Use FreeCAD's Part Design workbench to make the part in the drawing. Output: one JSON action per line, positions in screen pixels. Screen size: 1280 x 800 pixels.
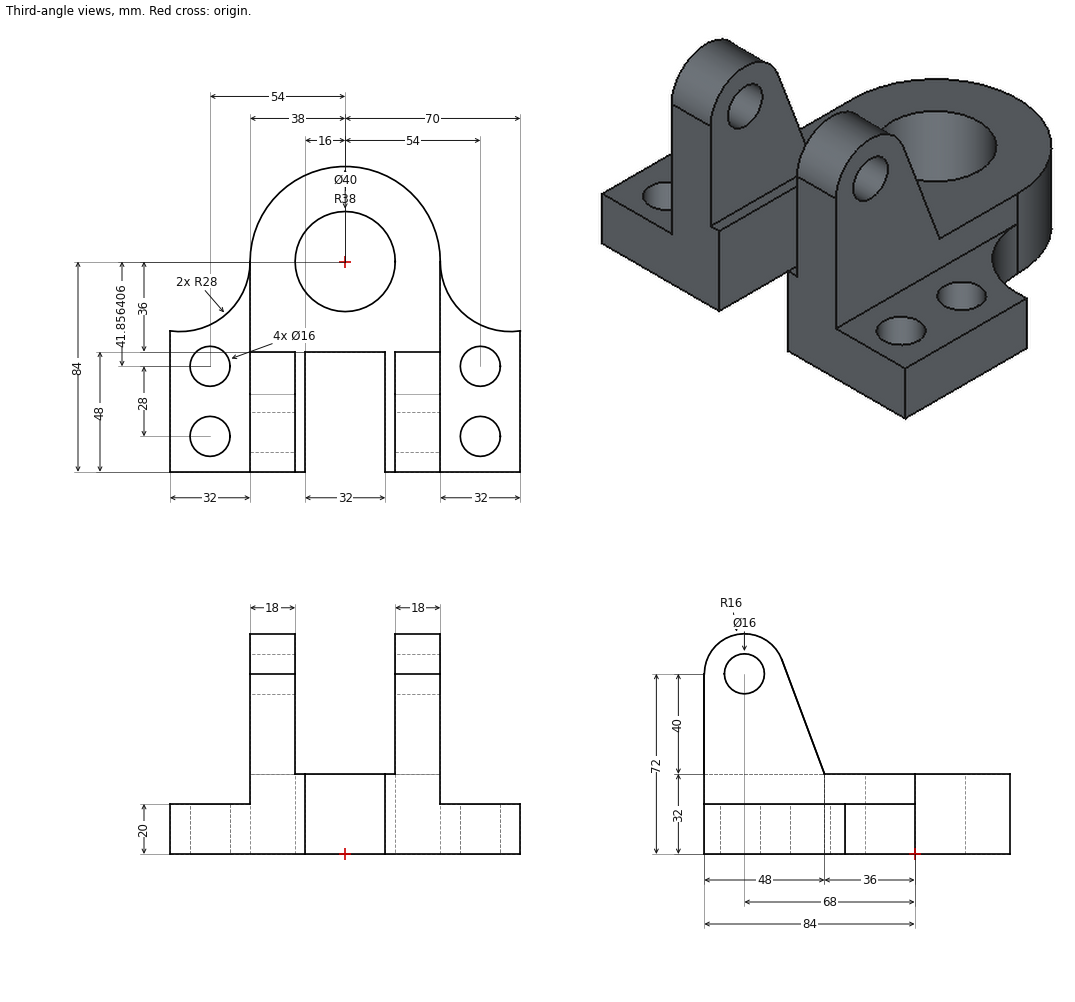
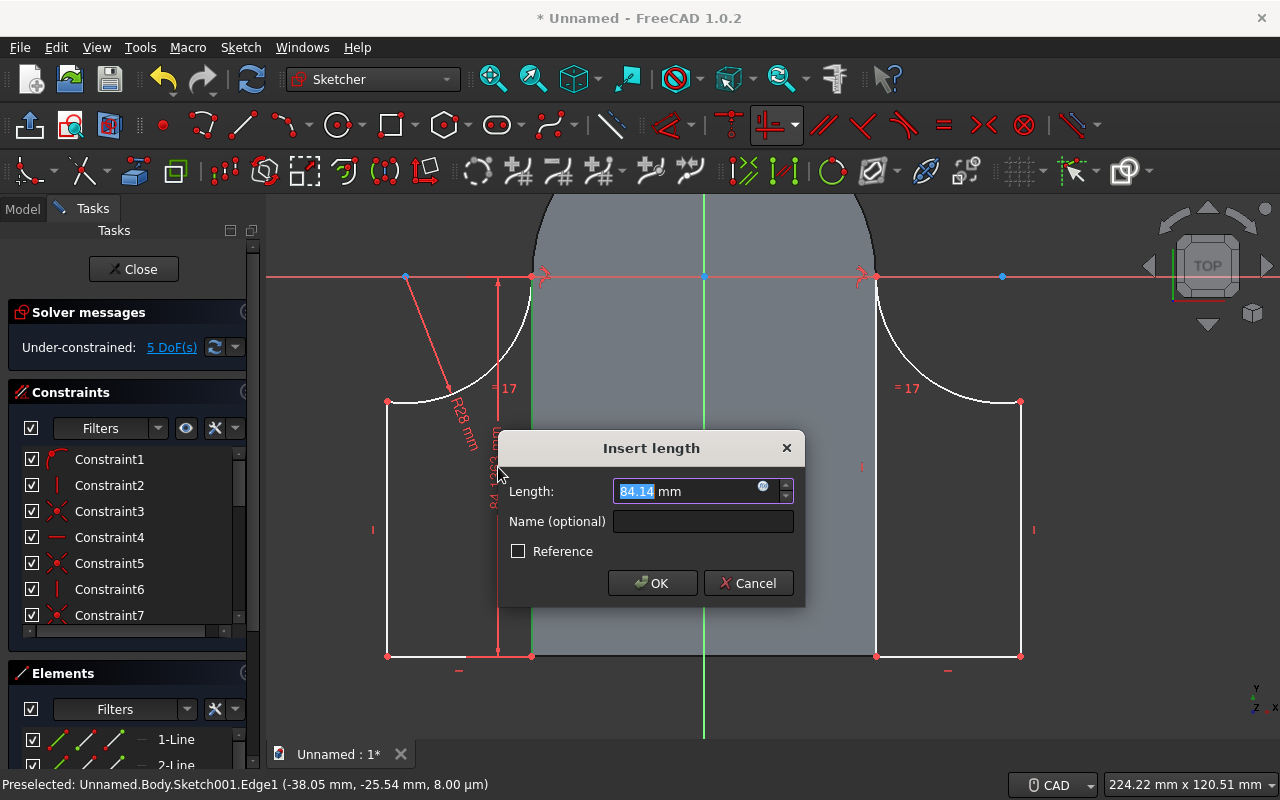
{"action": "type", "text": "84"}
{"action": "key", "text": "Return"}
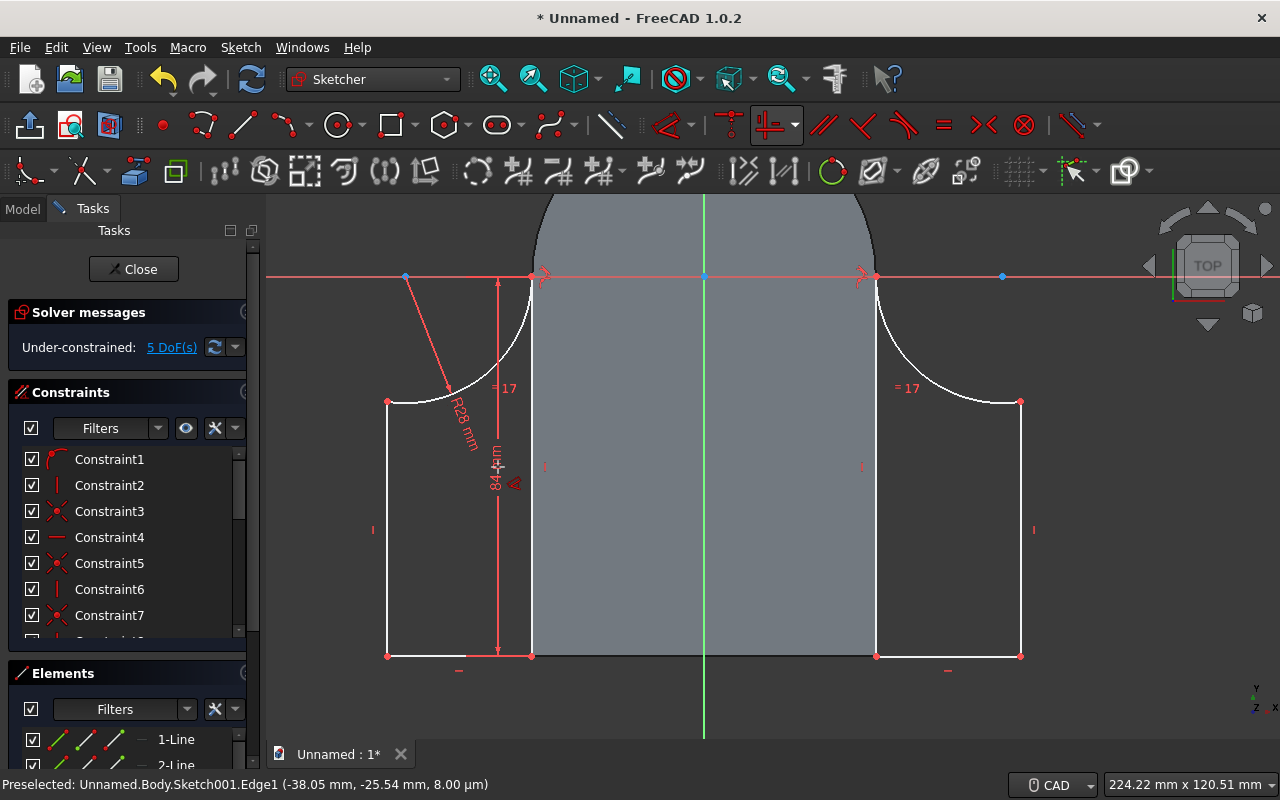
{"action": "left_click", "coordinate": [488, 656]}
{"action": "left_click", "coordinate": [459, 690]}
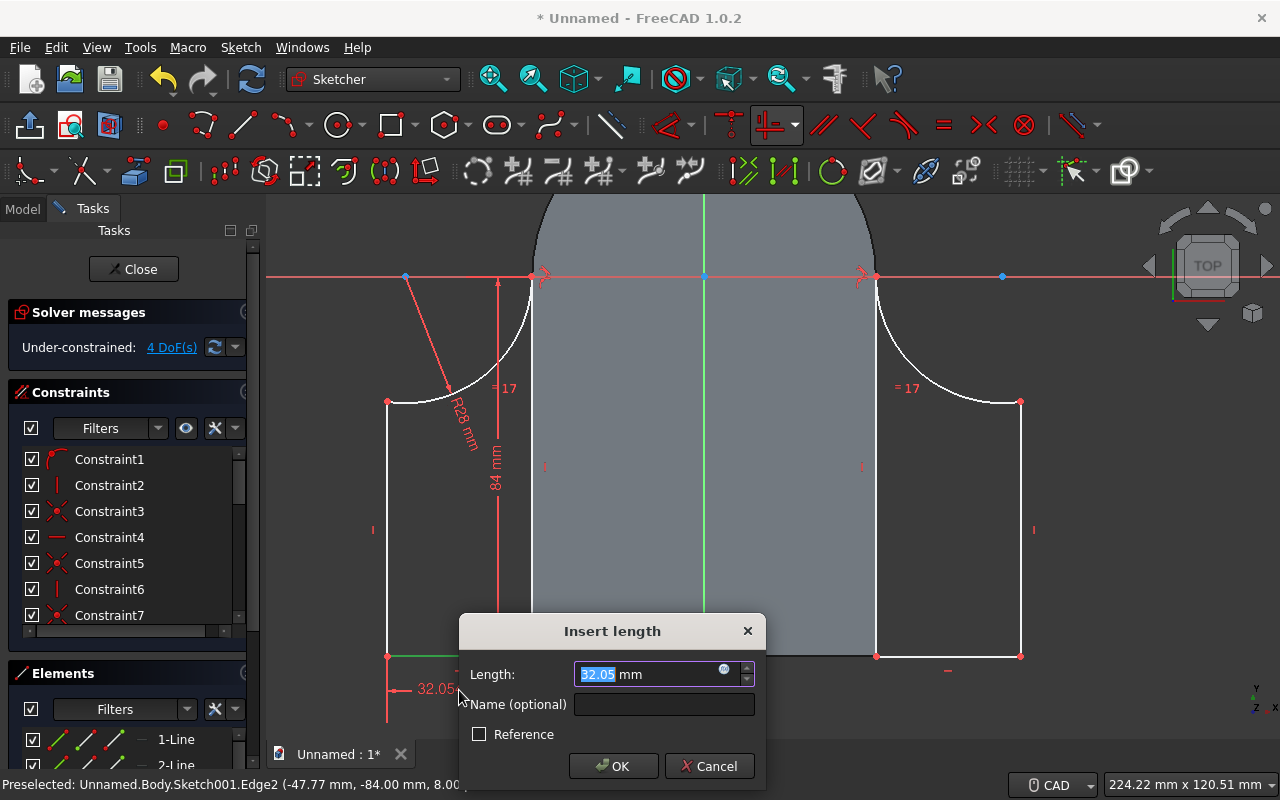
{"action": "type", "text": "32"}
{"action": "key", "text": "Return"}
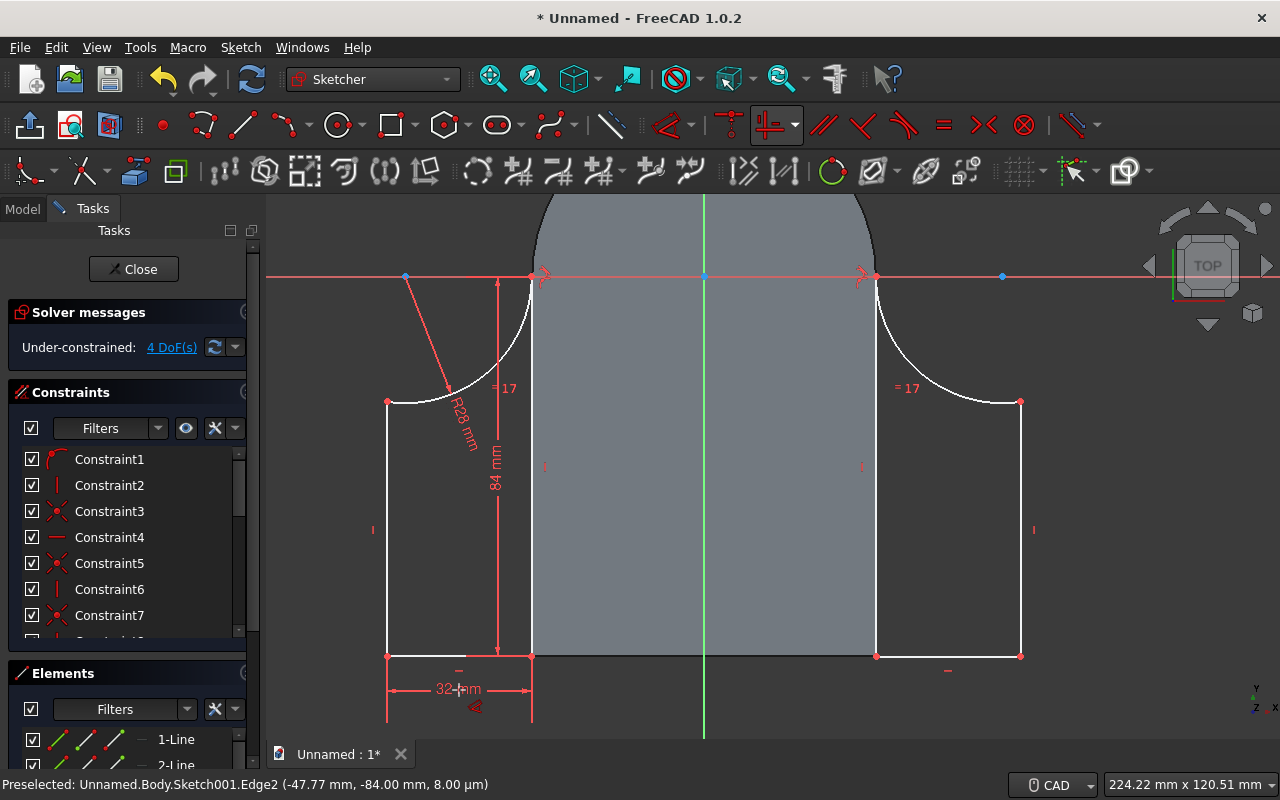
{"action": "left_click", "coordinate": [978, 657]}
{"action": "left_click", "coordinate": [949, 691]}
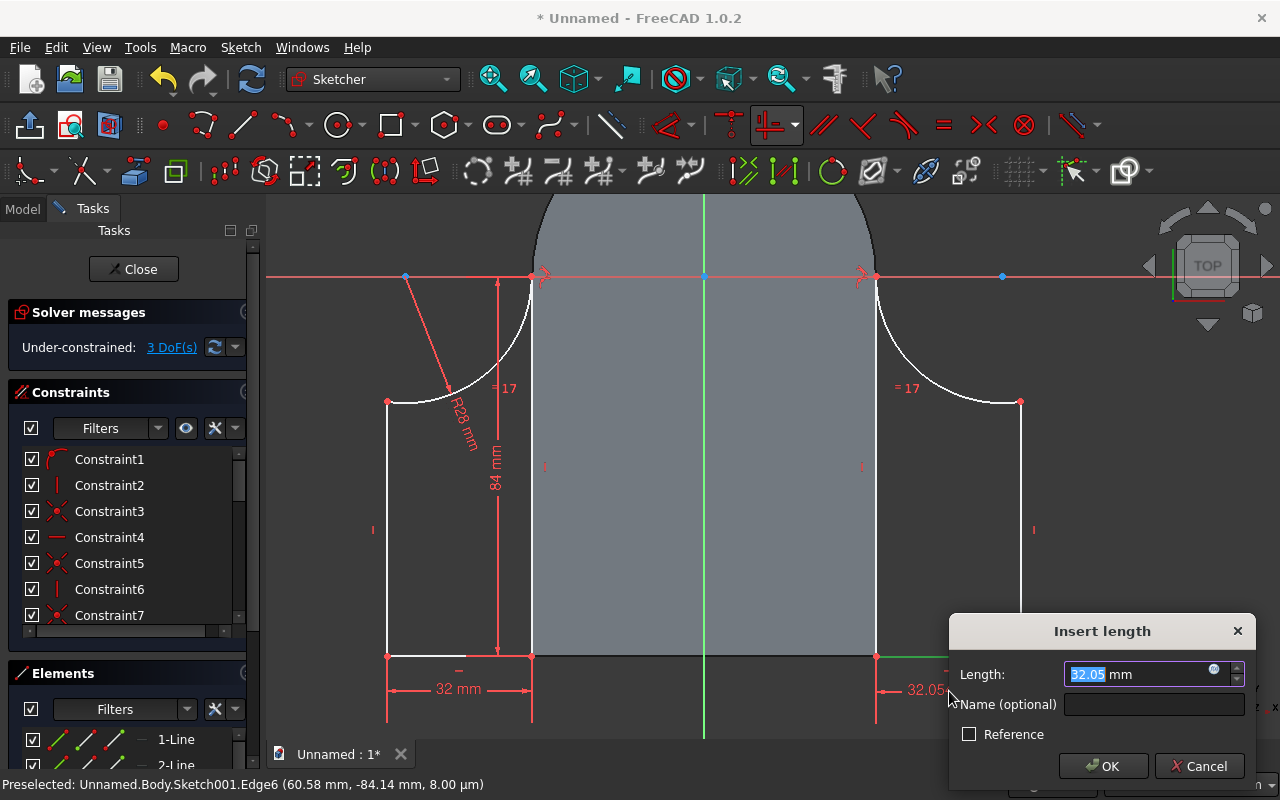
{"action": "type", "text": "32"}
{"action": "key", "text": "Return"}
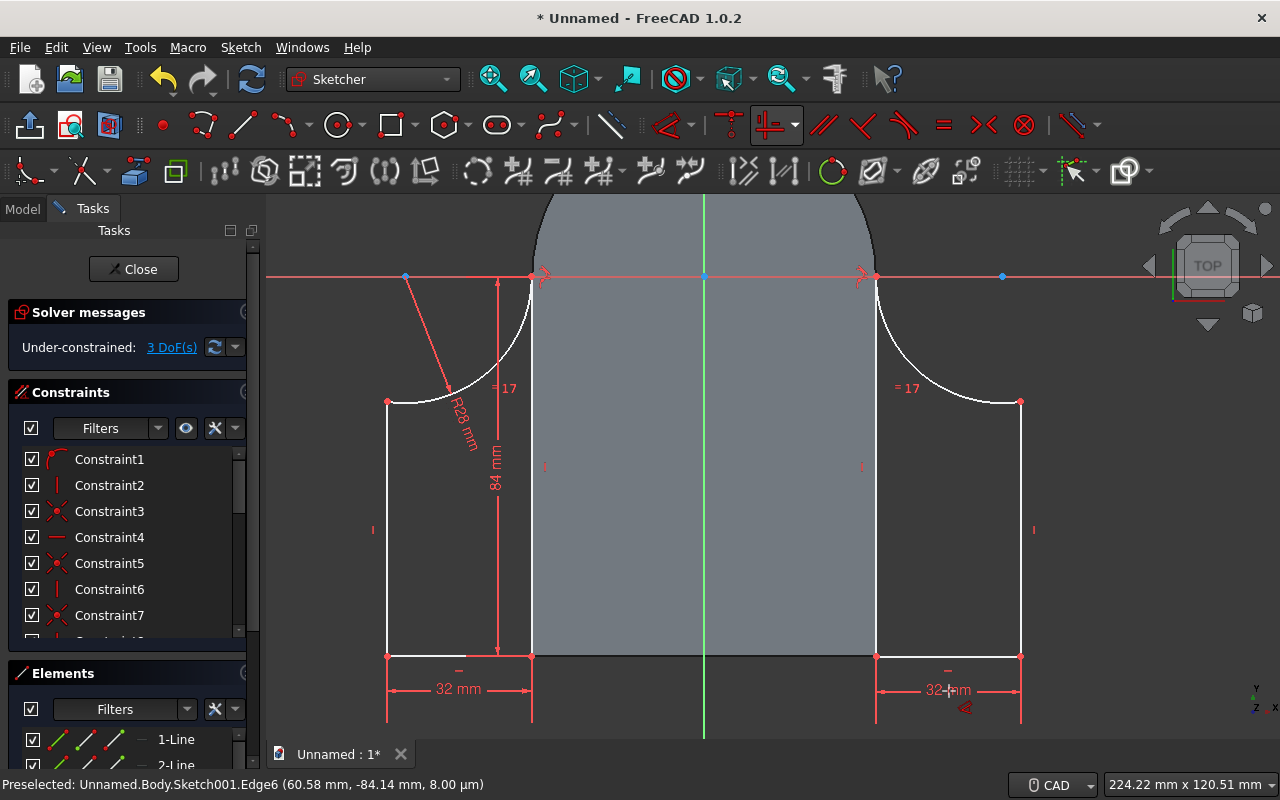
{"action": "left_click", "coordinate": [876, 543]}
{"action": "left_click", "coordinate": [910, 467]}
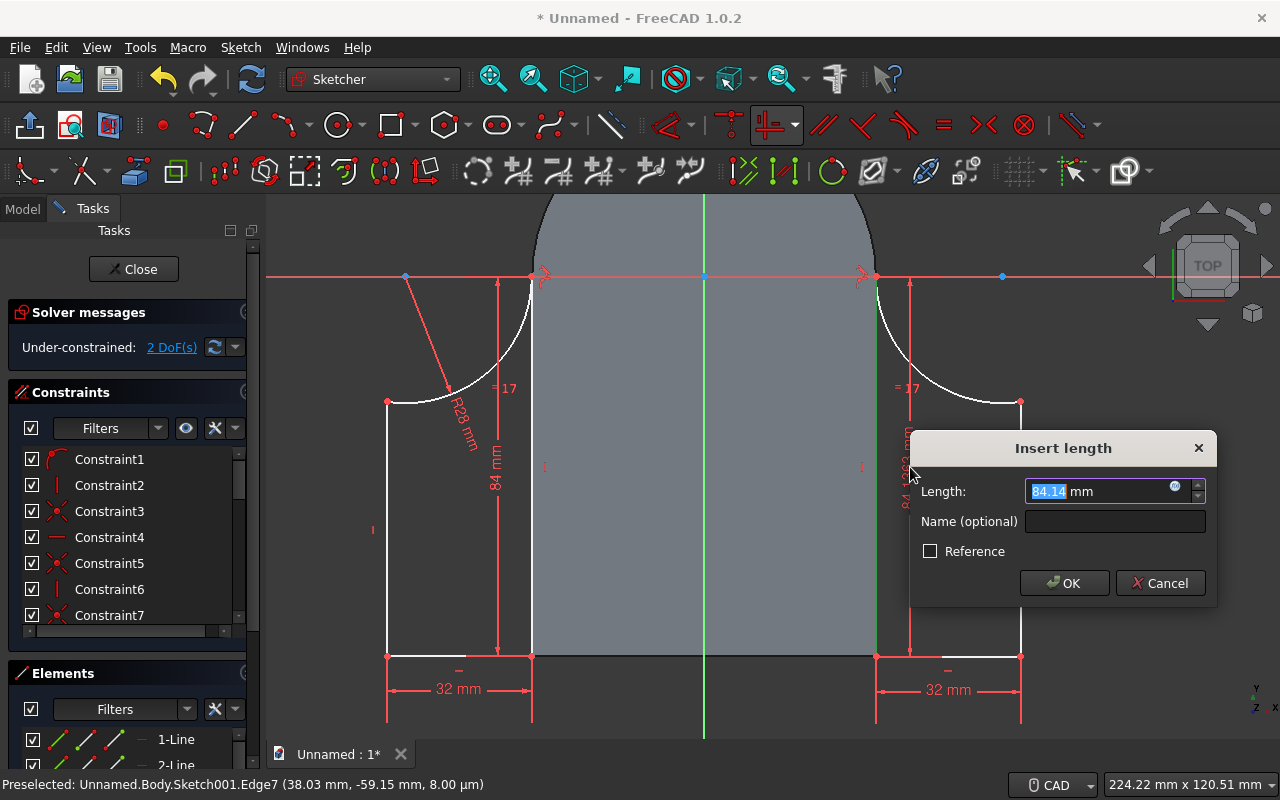
{"action": "type", "text": "84"}
{"action": "key", "text": "Return"}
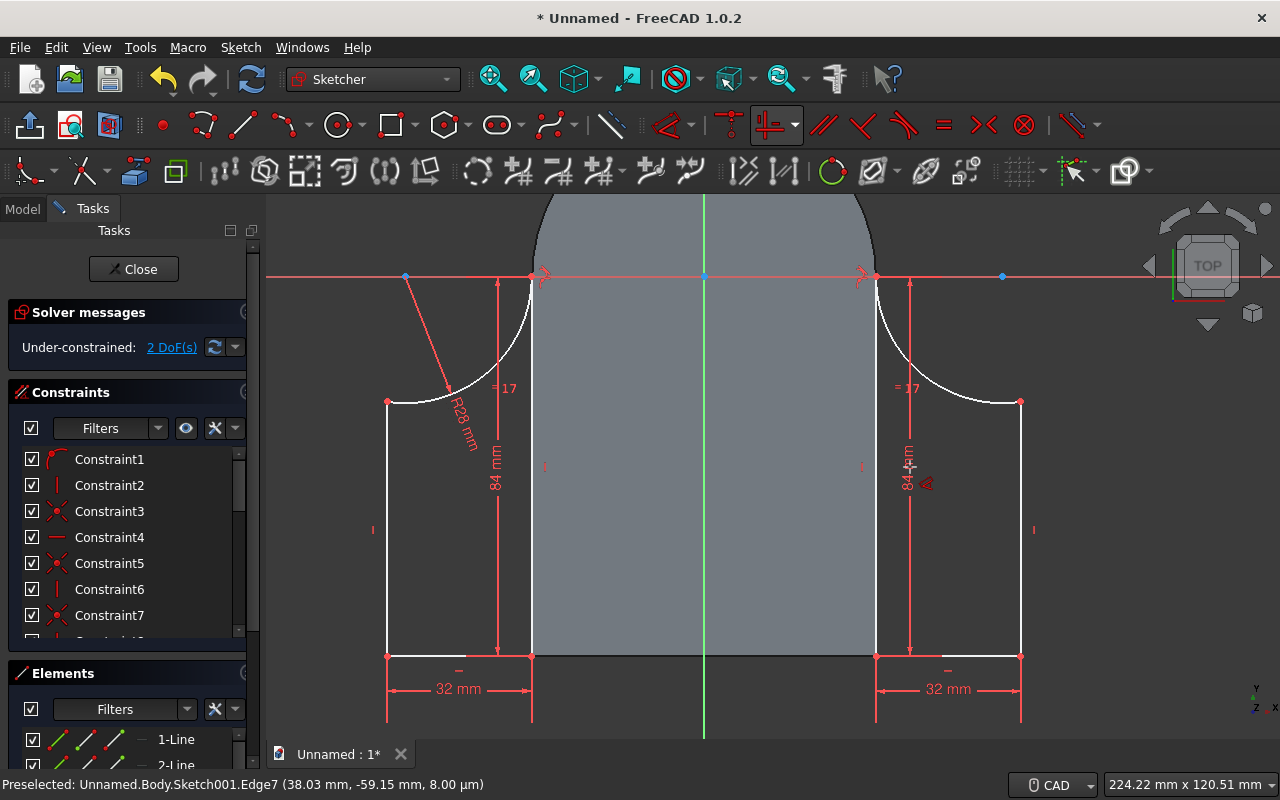
{"action": "left_click", "coordinate": [532, 277]}
{"action": "left_click", "coordinate": [618, 243]}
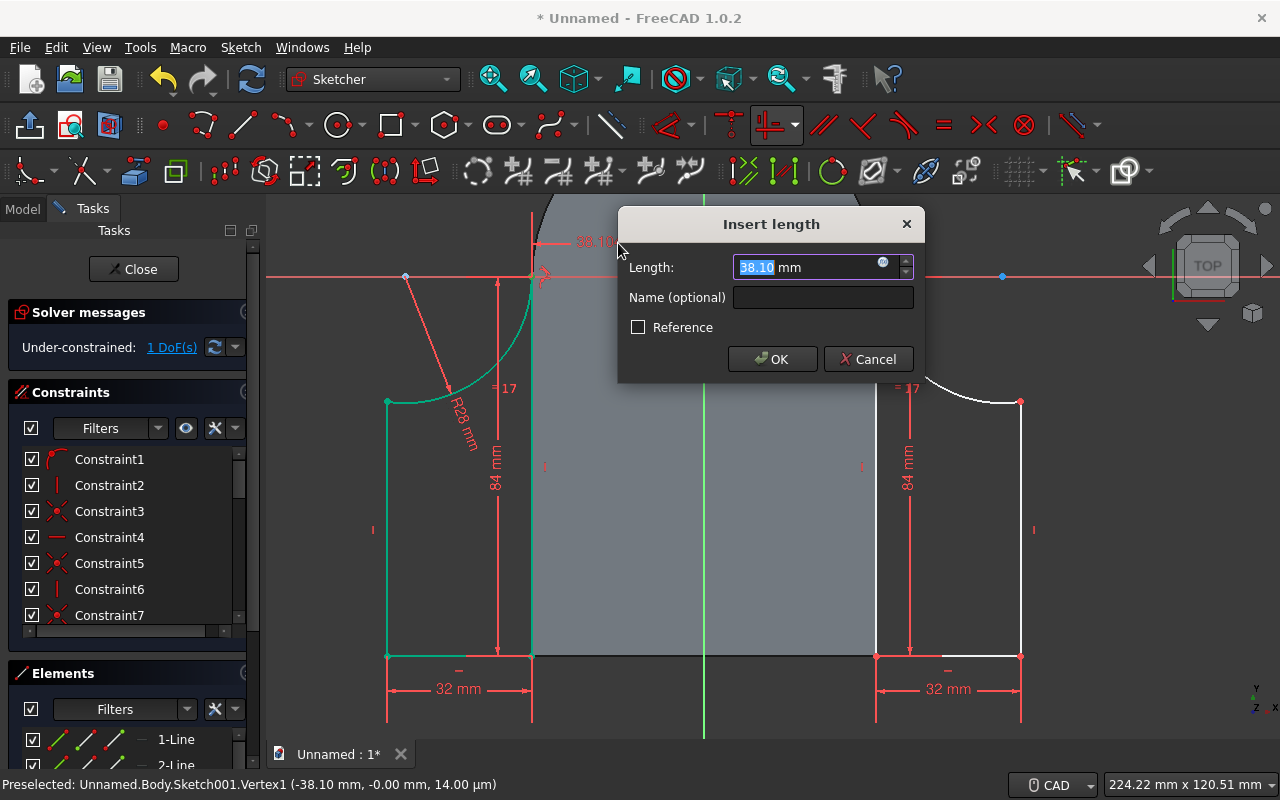
{"action": "type", "text": "38"}
{"action": "key", "text": "Return"}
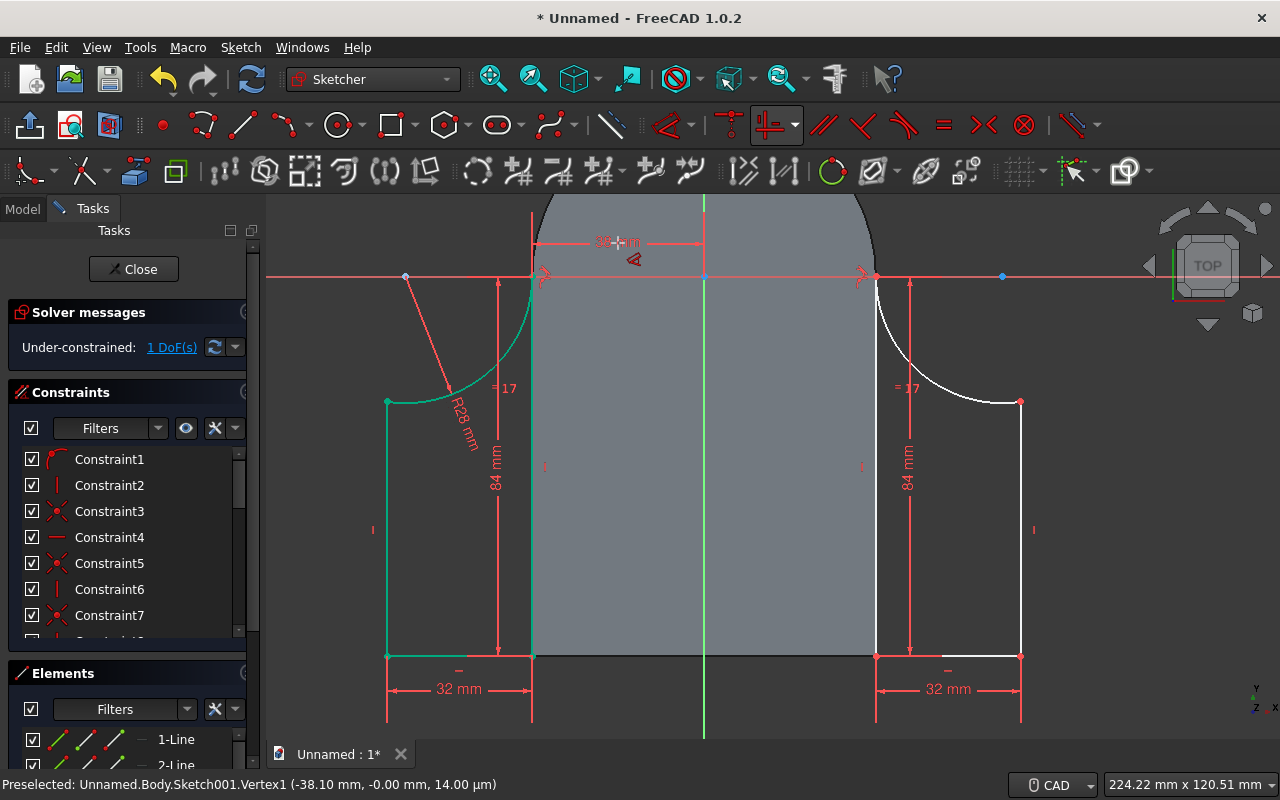
{"action": "left_click", "coordinate": [1021, 402]}
{"action": "left_click", "coordinate": [862, 243]}